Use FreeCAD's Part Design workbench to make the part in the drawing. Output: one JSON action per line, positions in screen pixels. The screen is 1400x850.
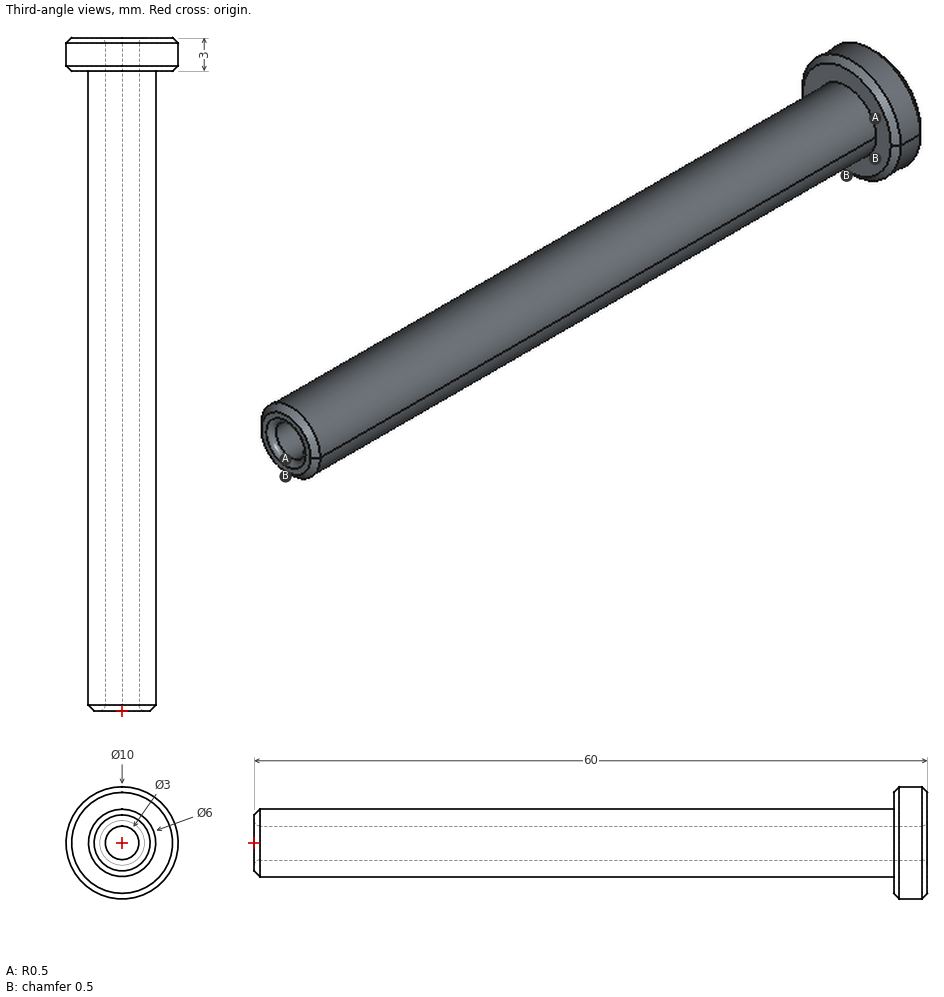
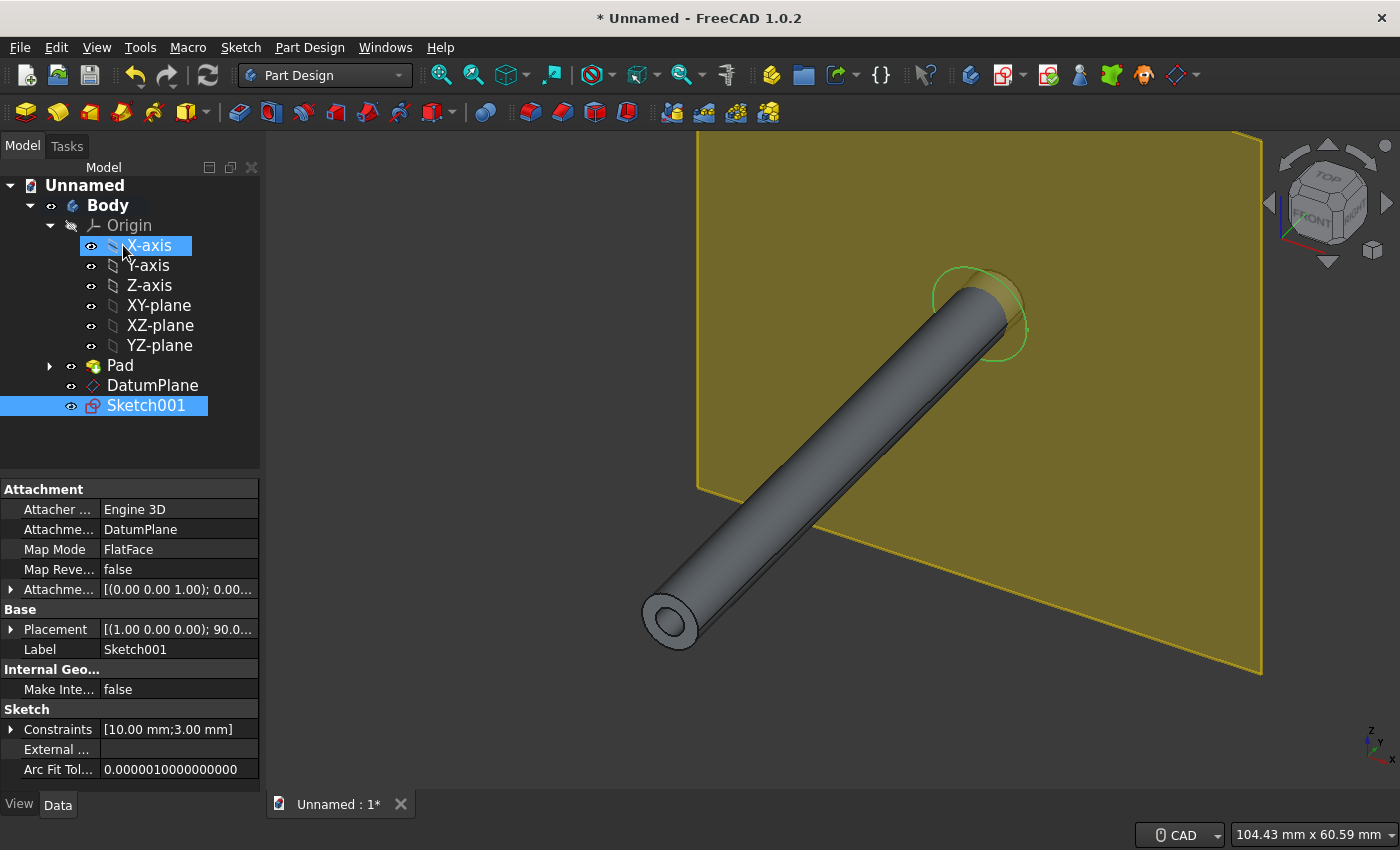
{"action": "left_click", "coordinate": [26, 112]}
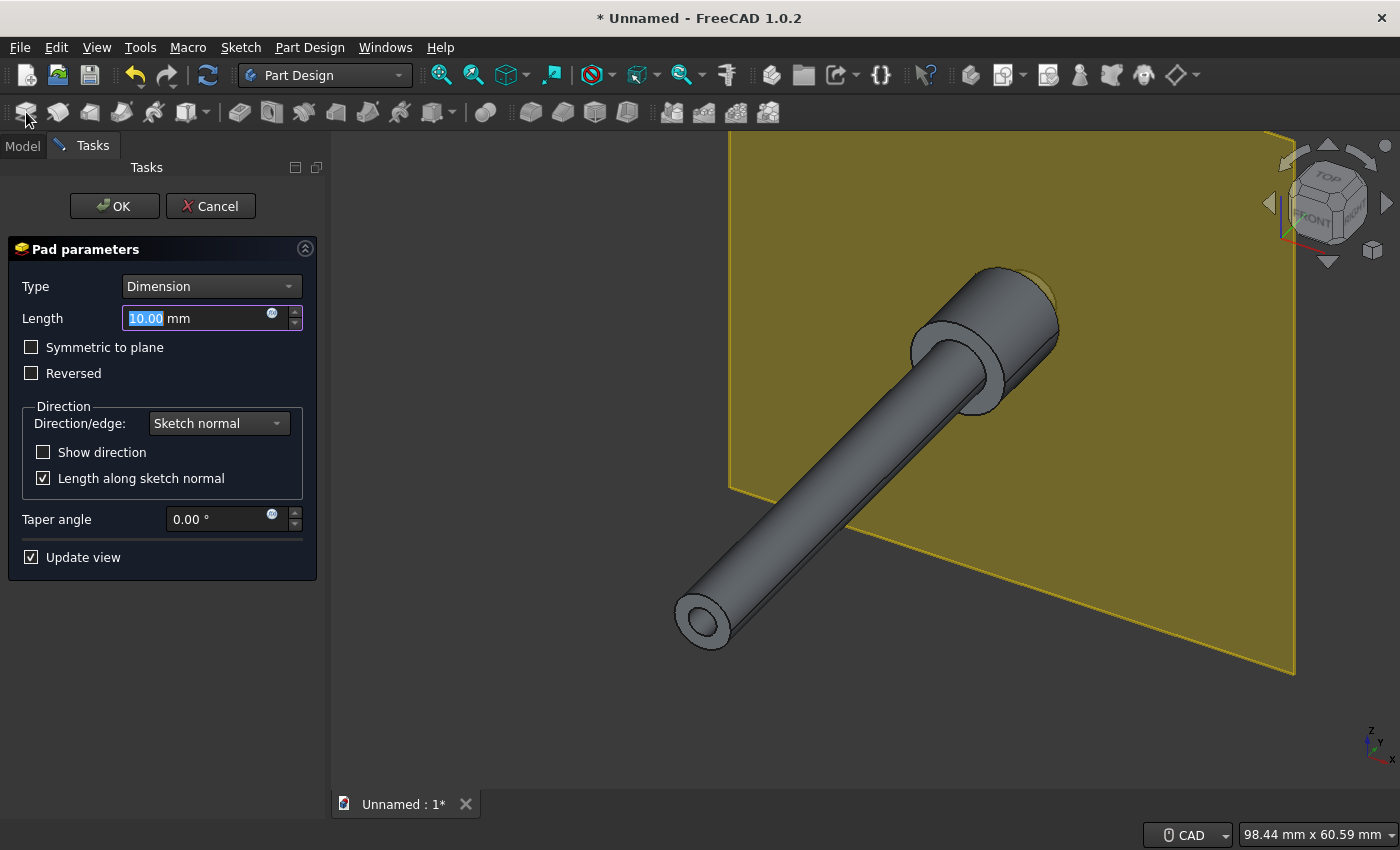
{"action": "type", "text": "3"}
{"action": "key", "text": "Tab"}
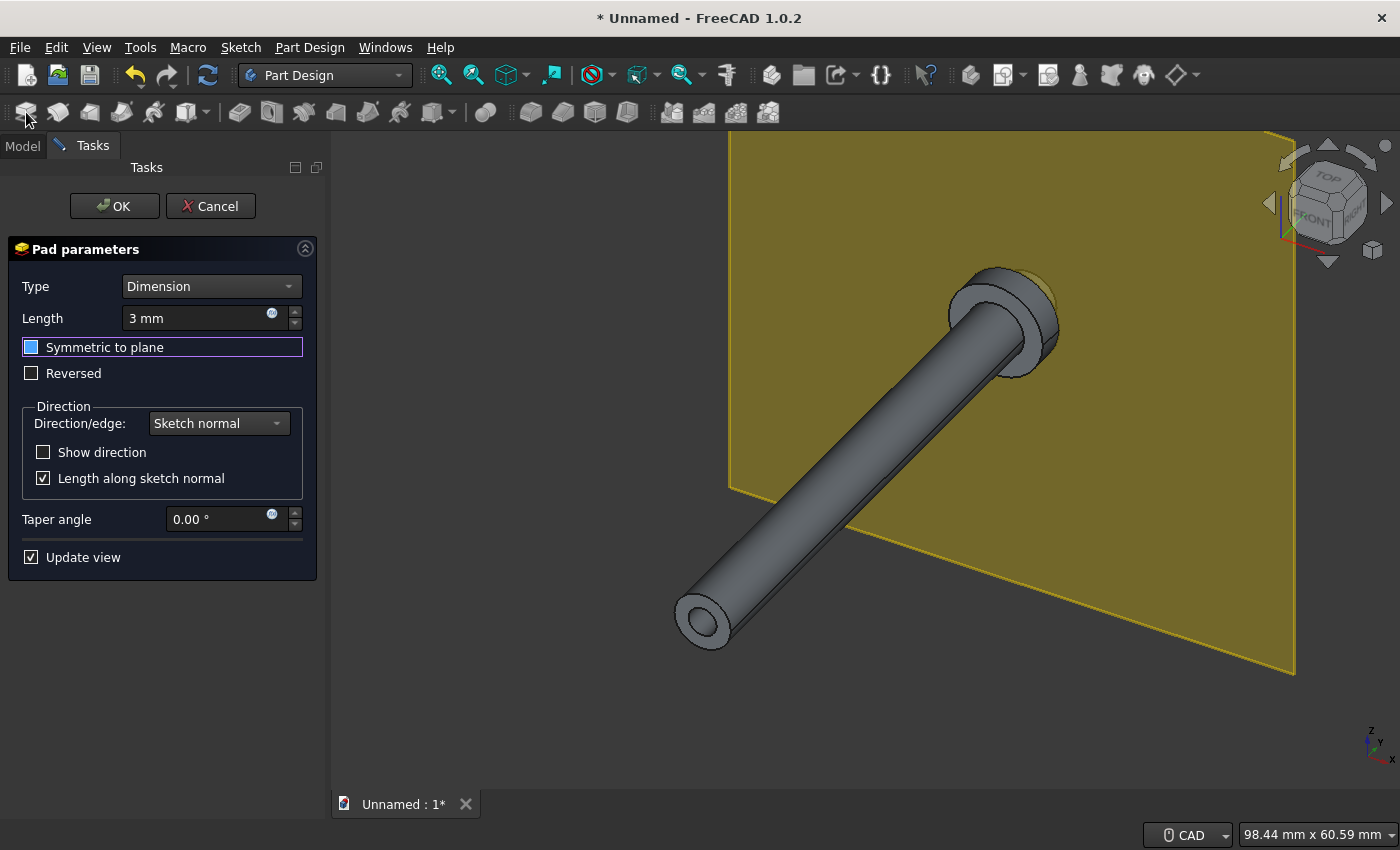
{"action": "left_click", "coordinate": [30, 373]}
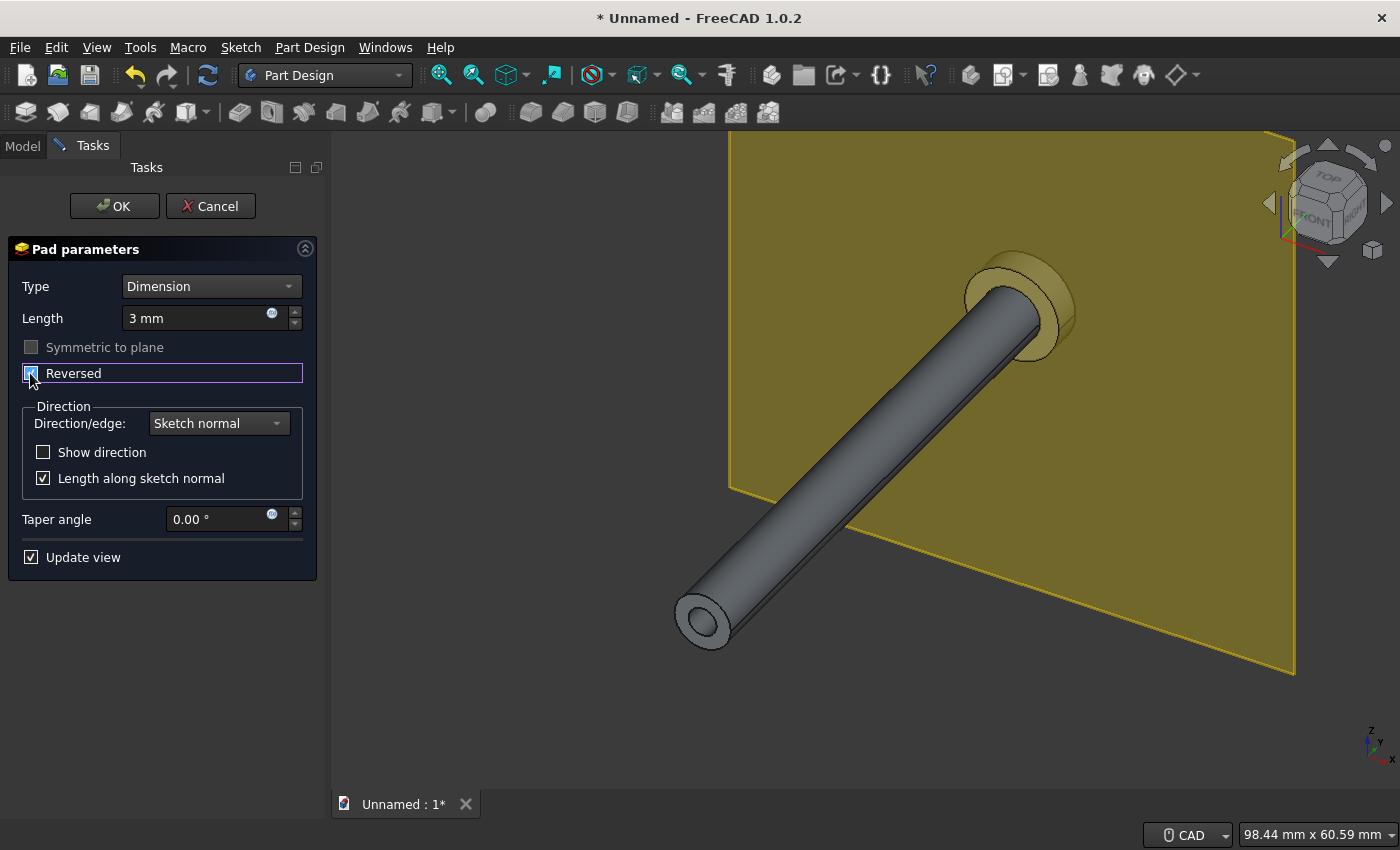
{"action": "left_click", "coordinate": [115, 206]}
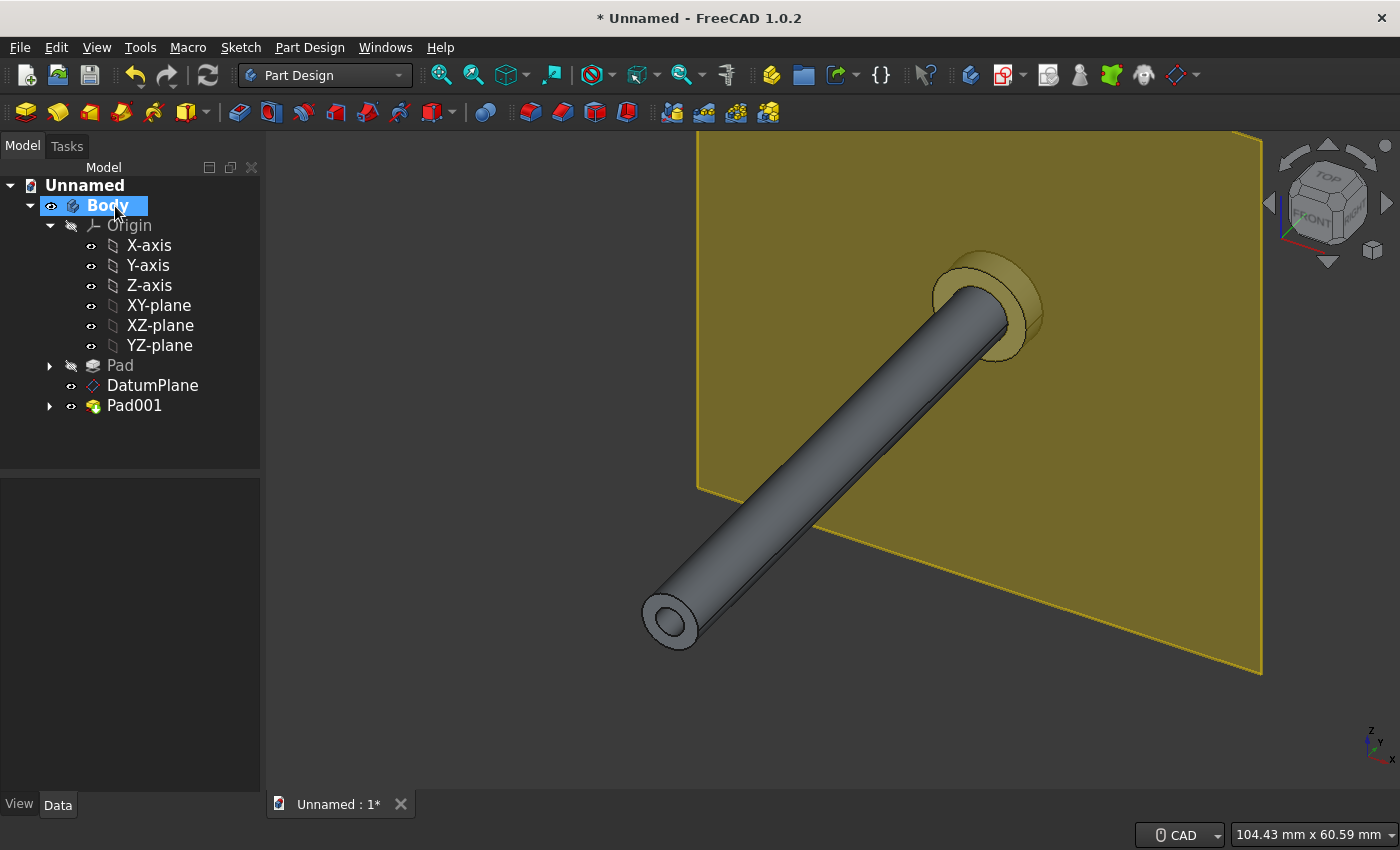
{"action": "left_click", "coordinate": [116, 386]}
{"action": "key", "text": "space"}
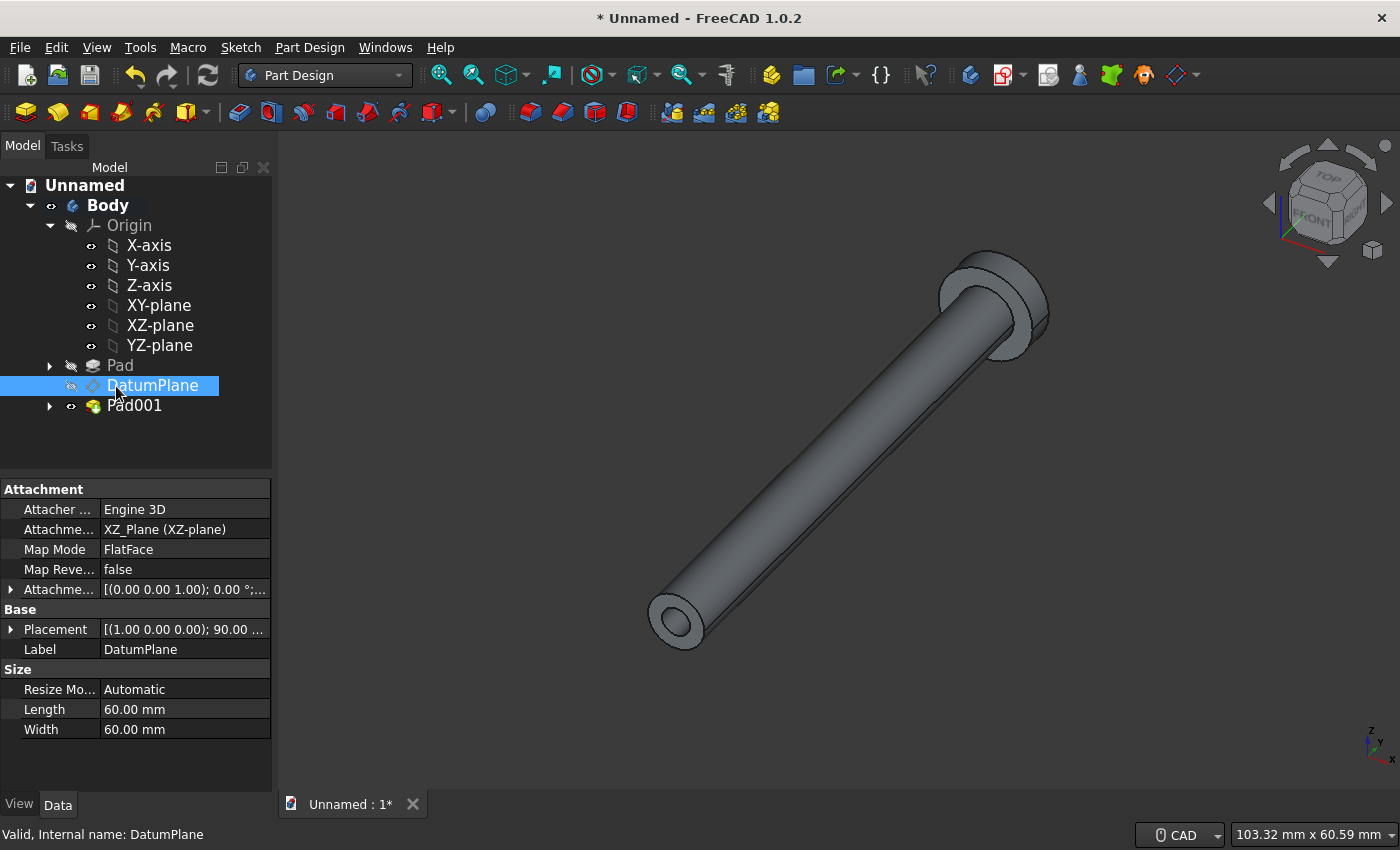
{"action": "left_click", "coordinate": [662, 616]}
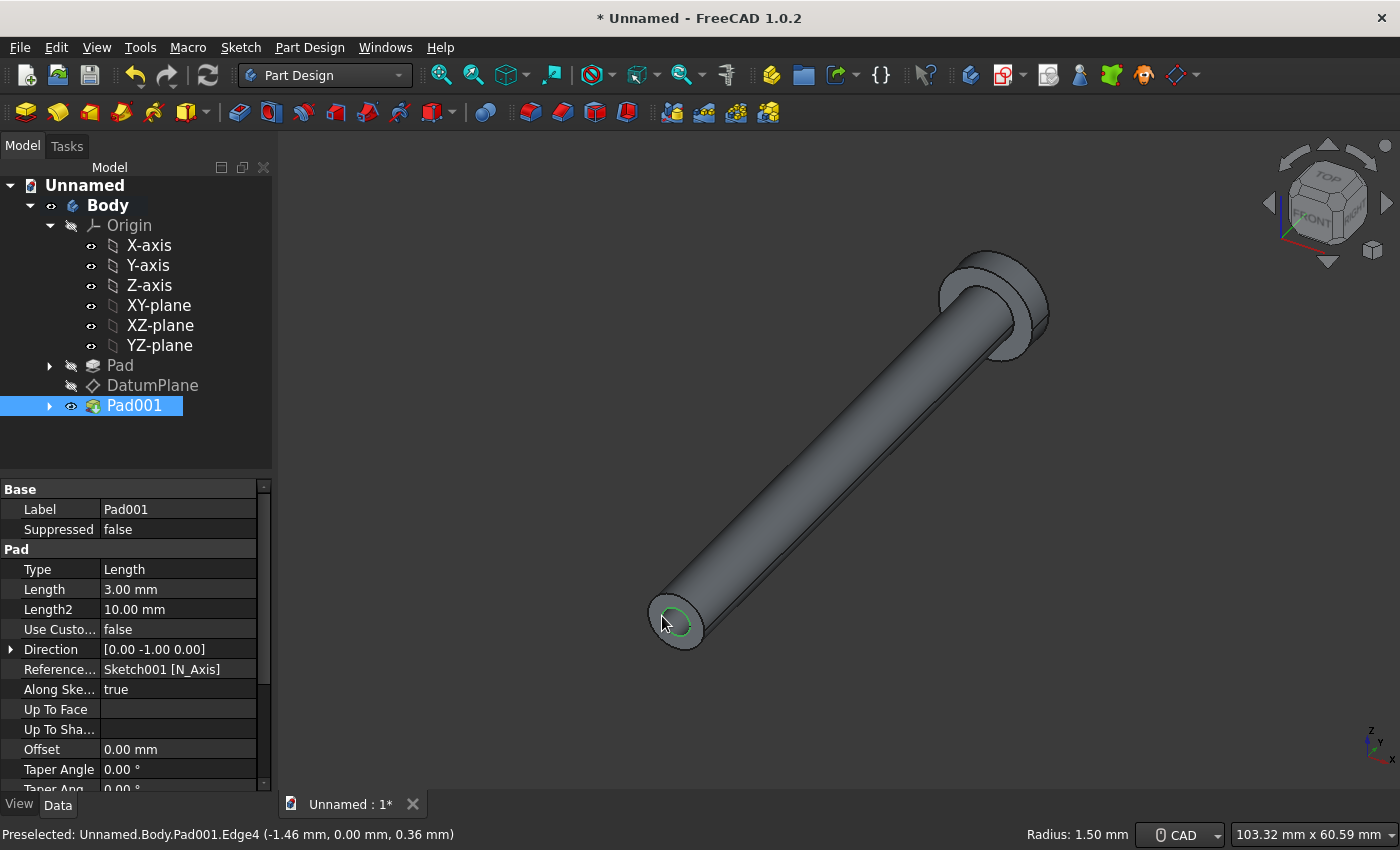
{"action": "key", "text": "0"}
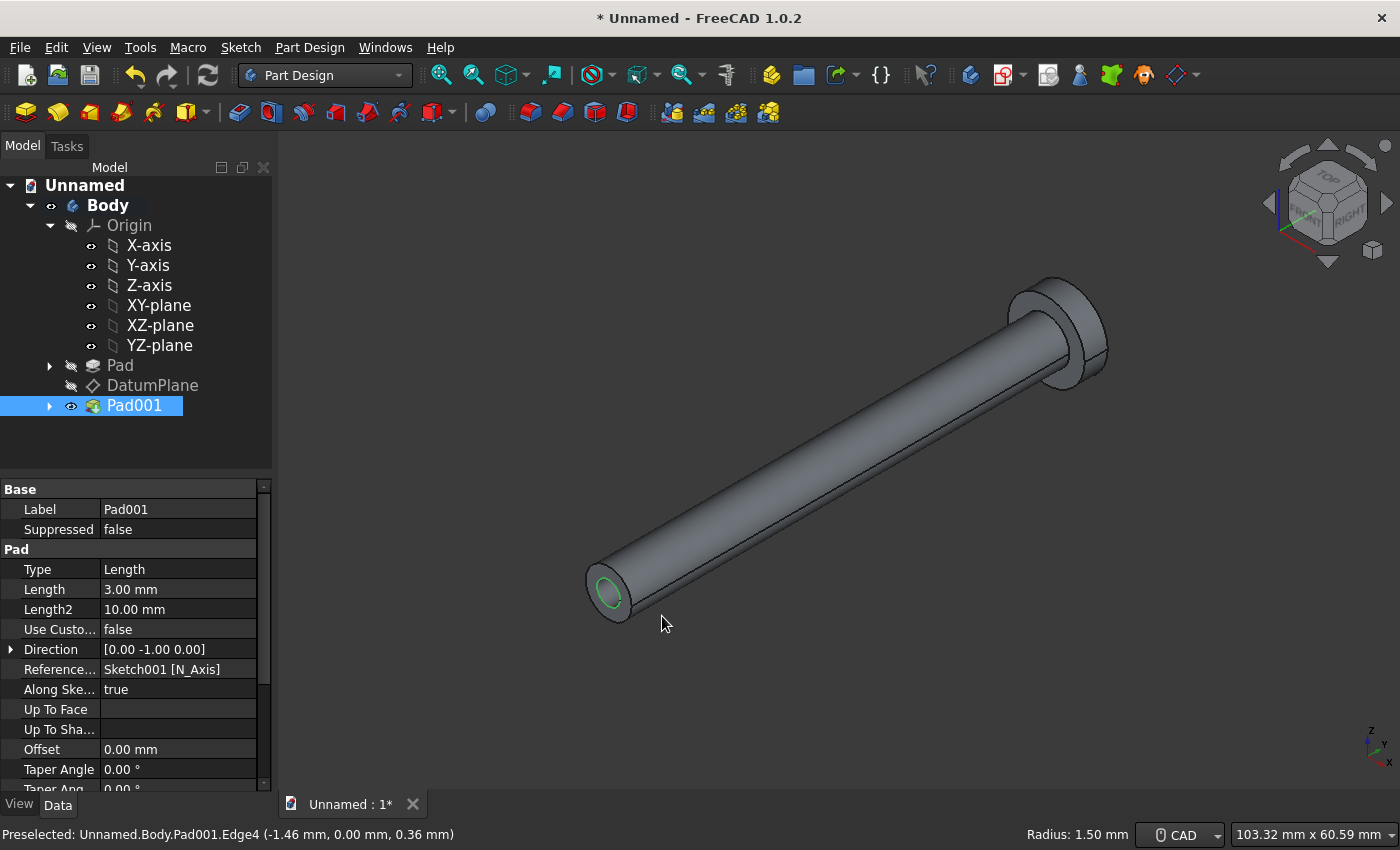
{"action": "key", "text": "2"}